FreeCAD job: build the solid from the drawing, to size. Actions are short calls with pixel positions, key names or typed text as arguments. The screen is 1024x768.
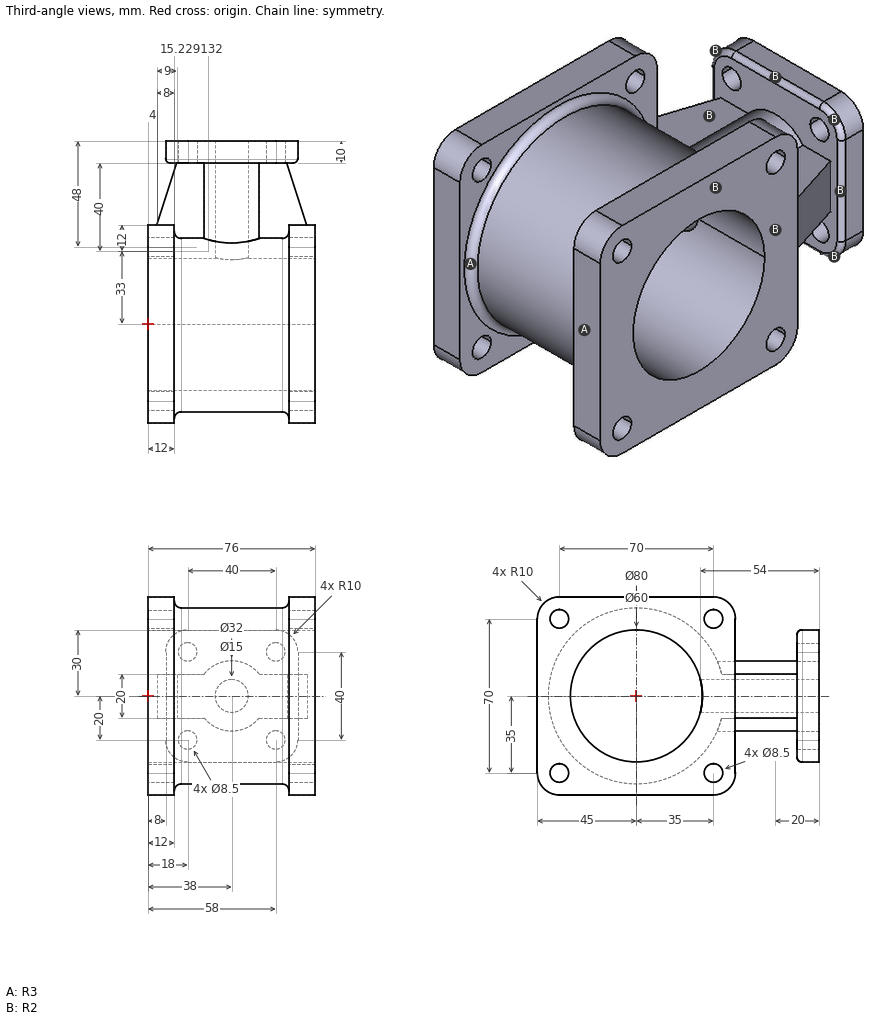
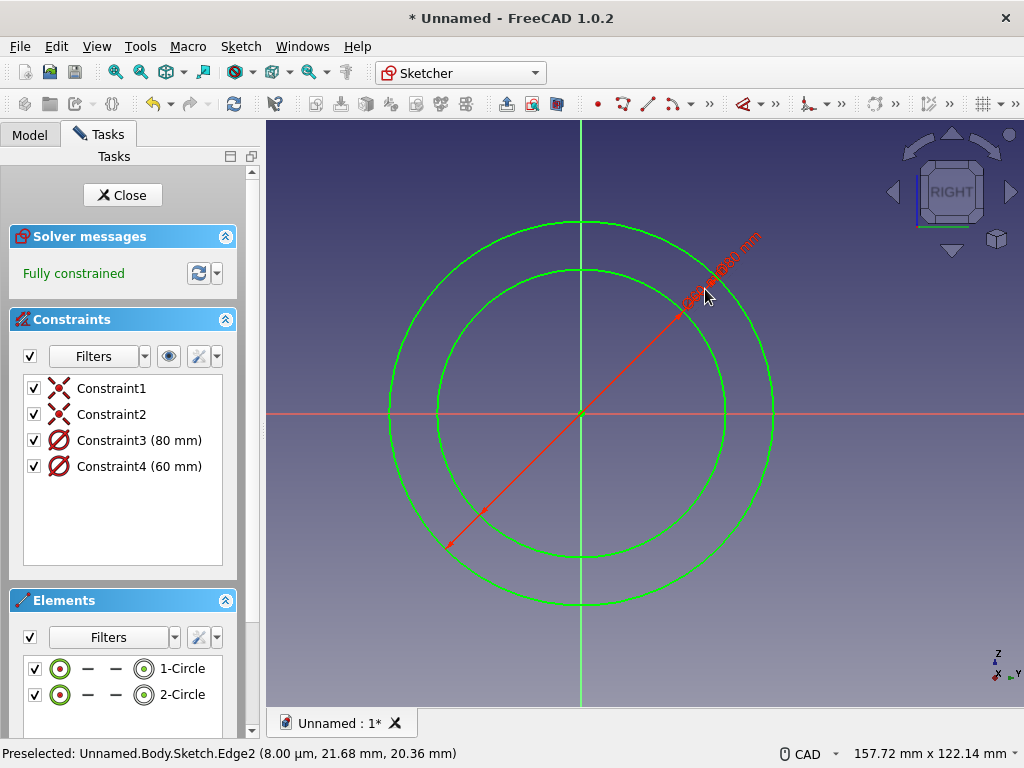
click(123, 195)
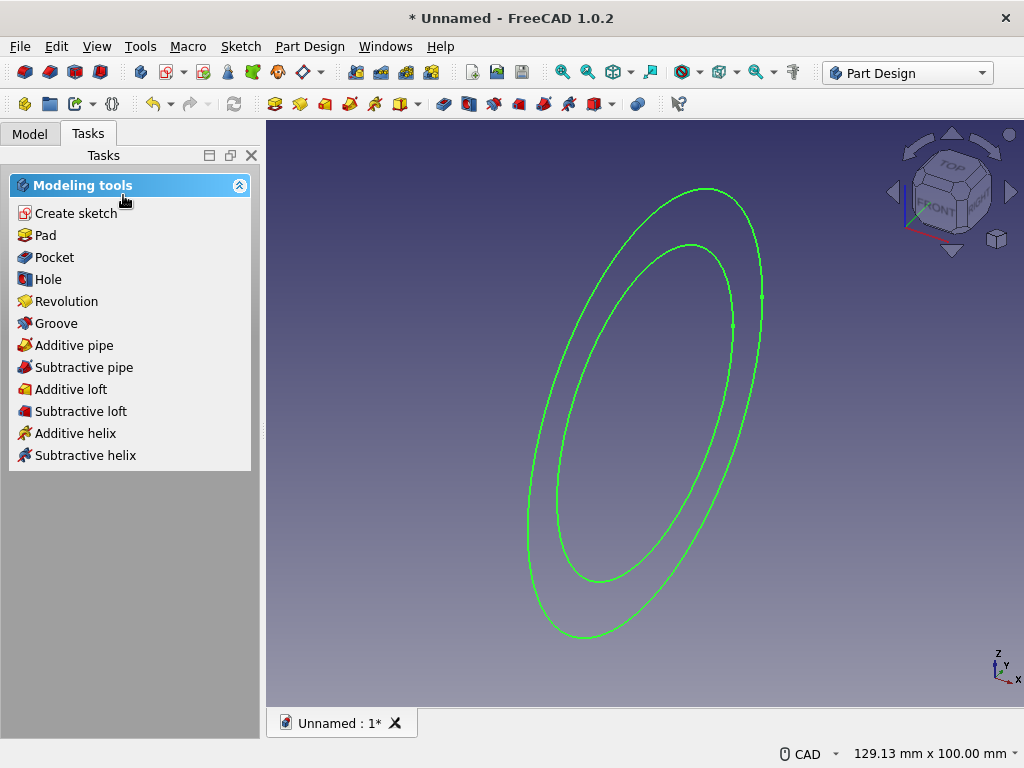
click(275, 104)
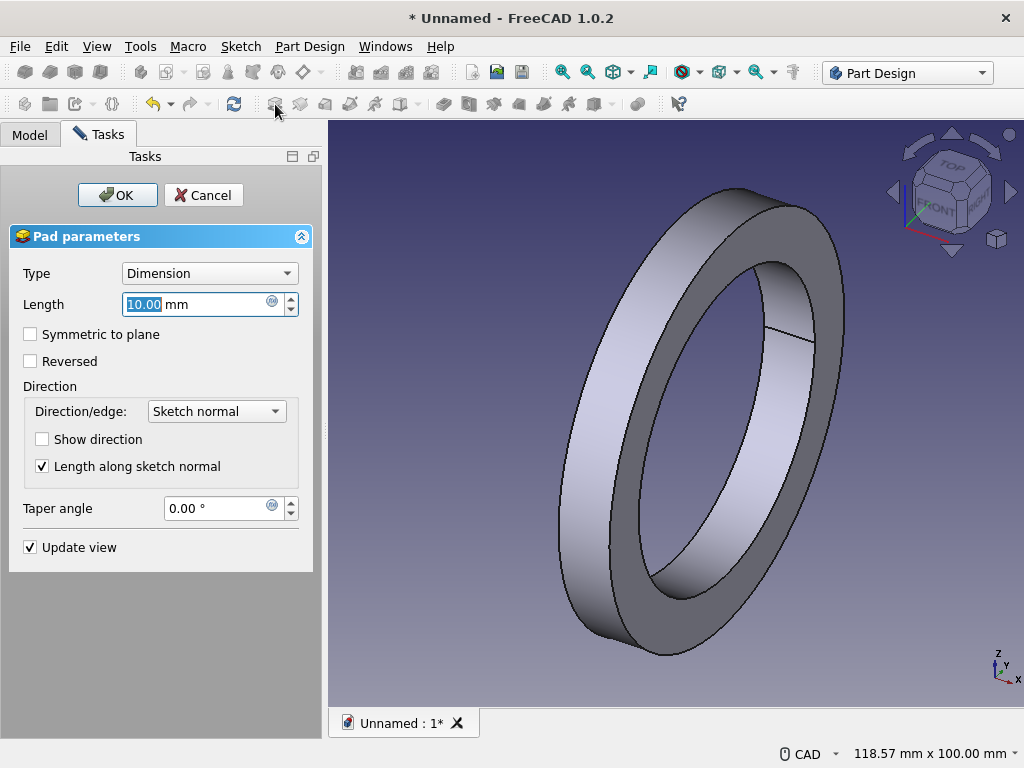
text(76)
key(Tab)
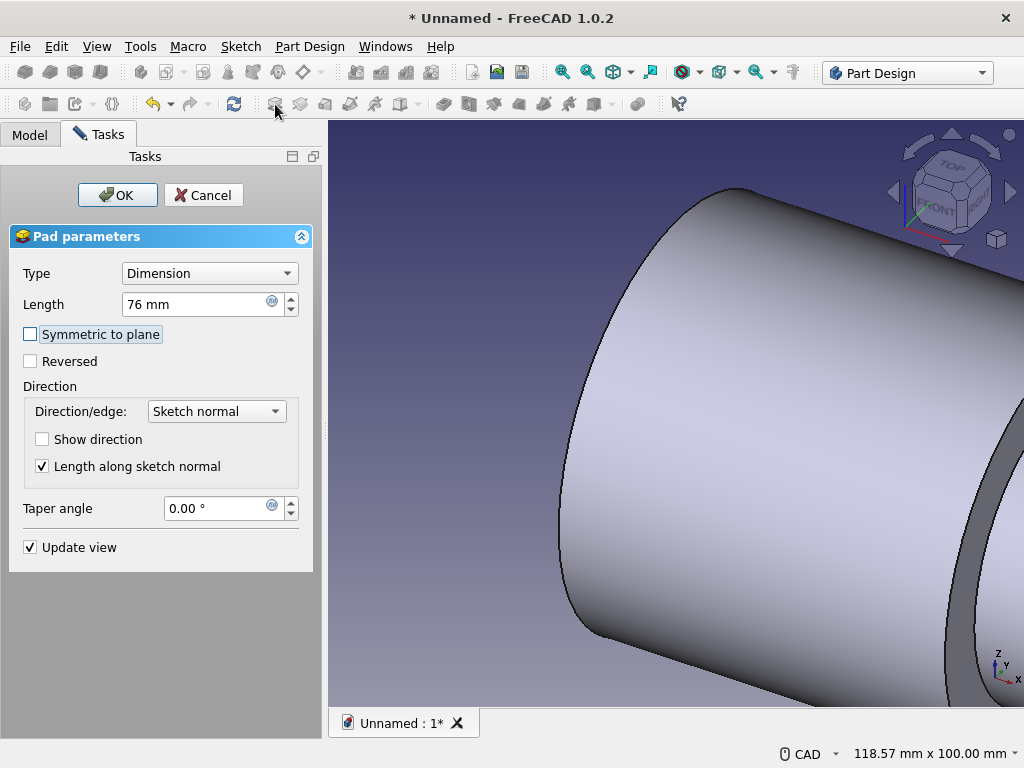
click(118, 195)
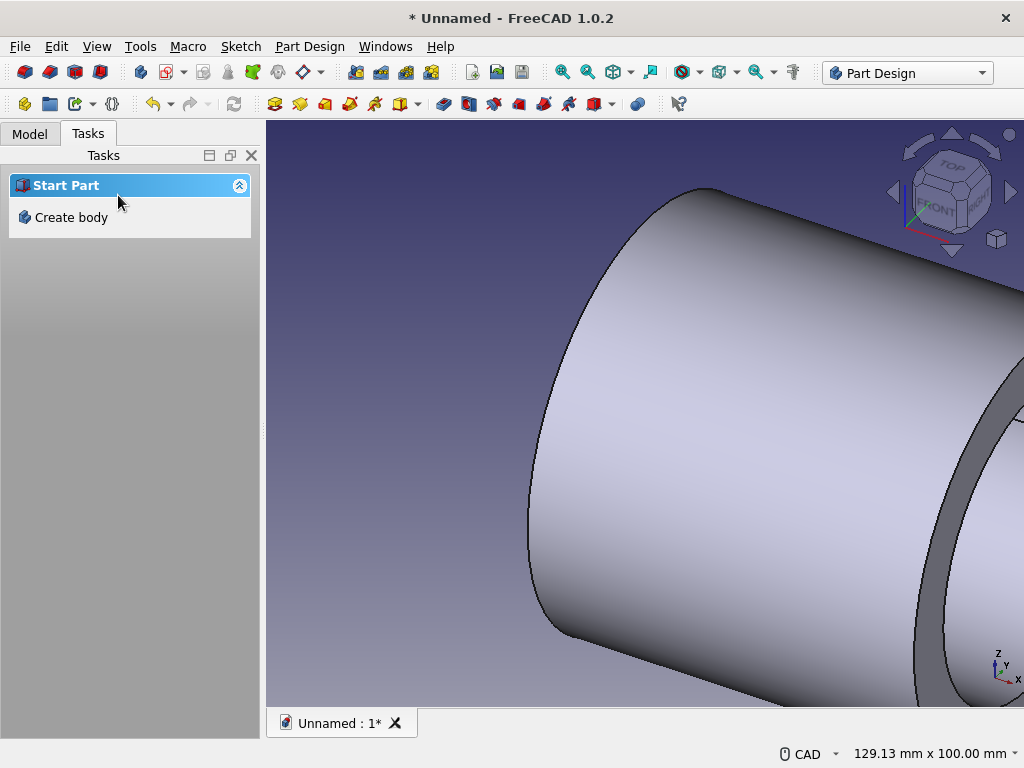
key(v)
key(f)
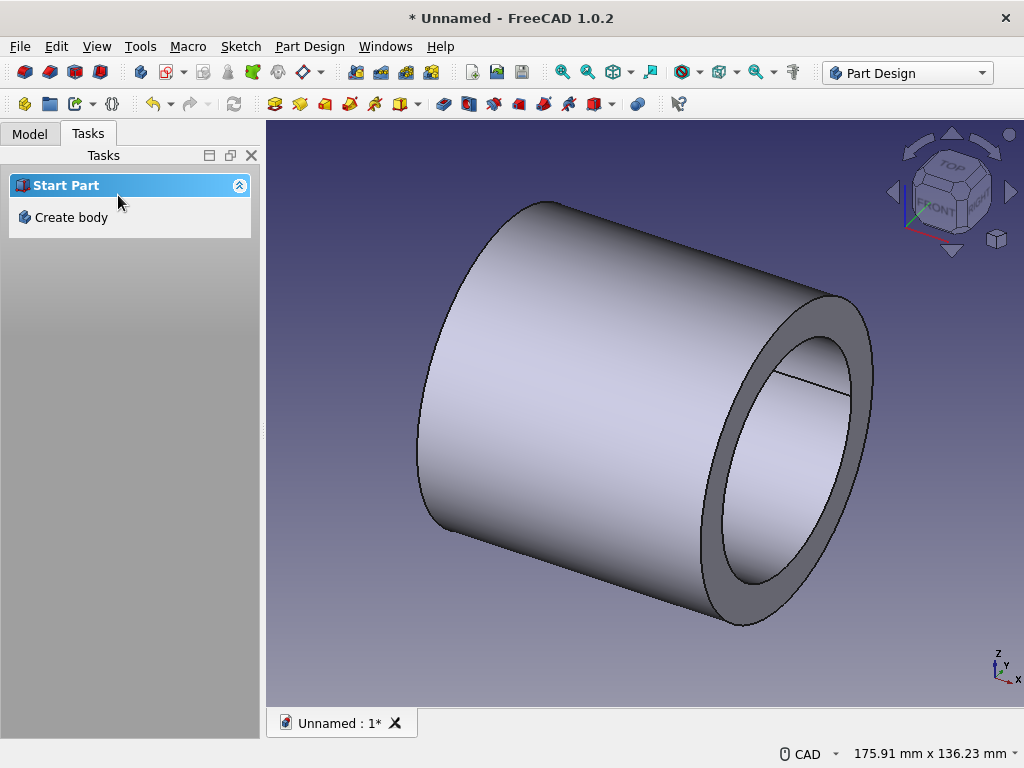
click(166, 72)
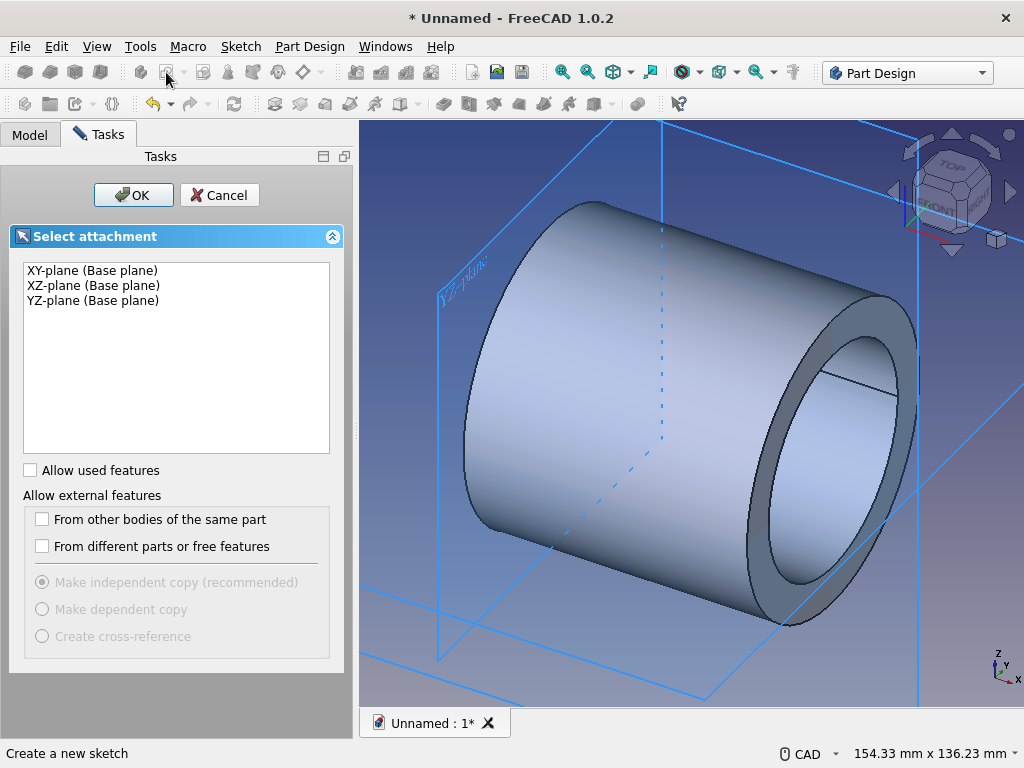
click(84, 300)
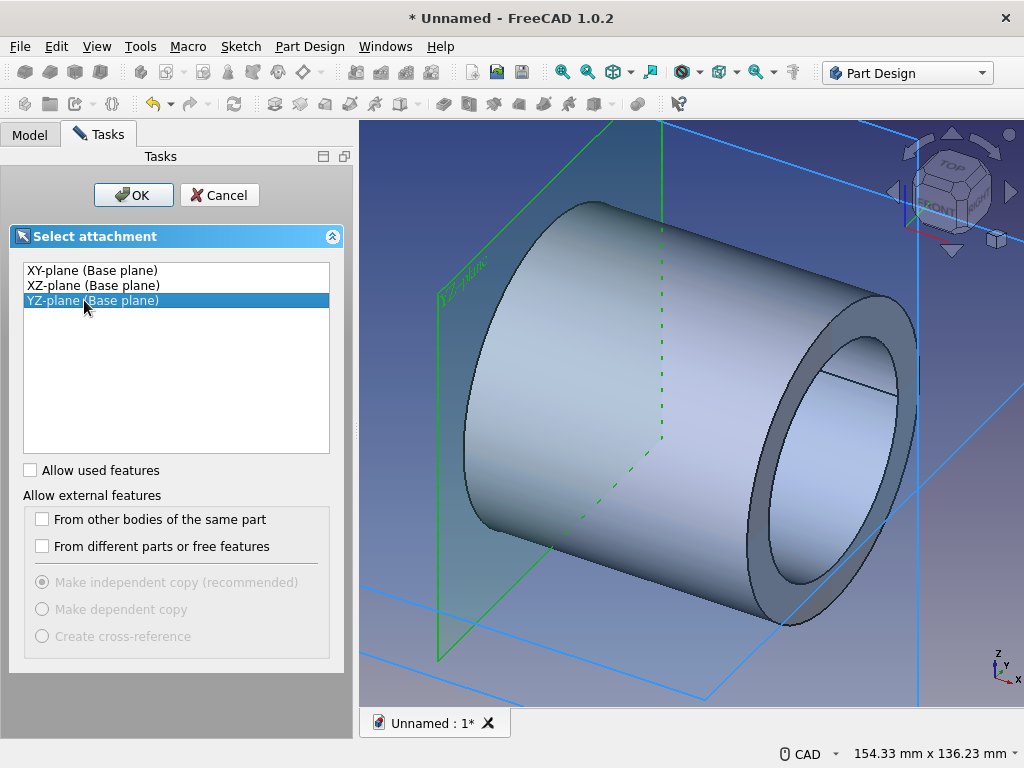
click(134, 195)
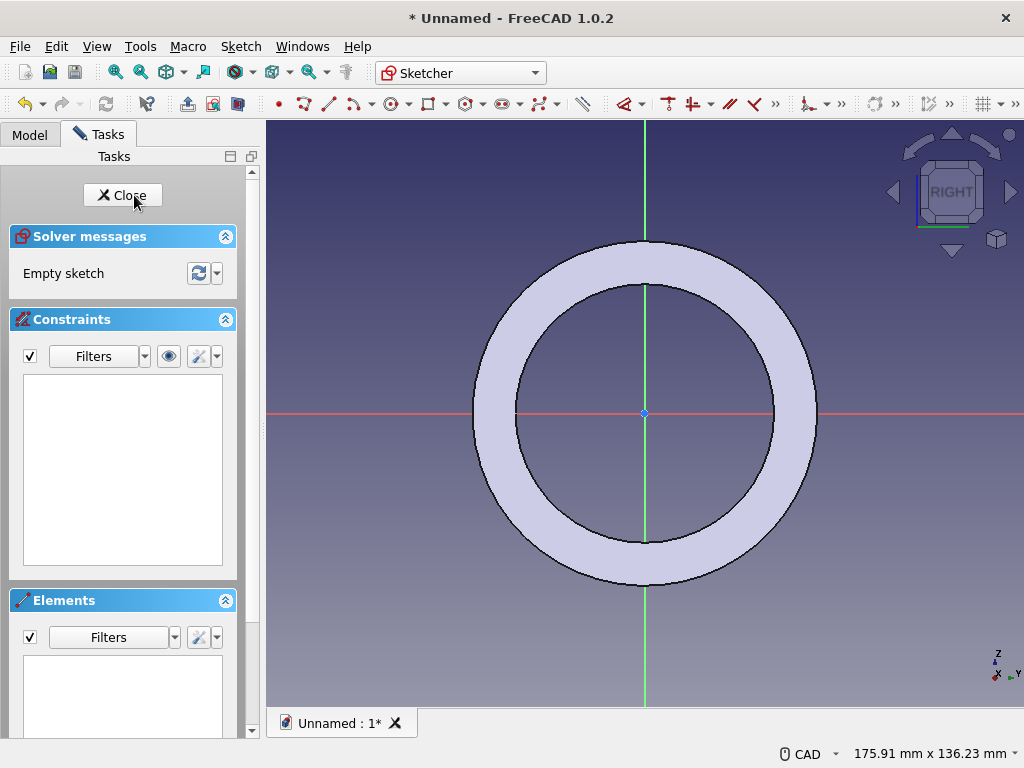
key(q)
key(s)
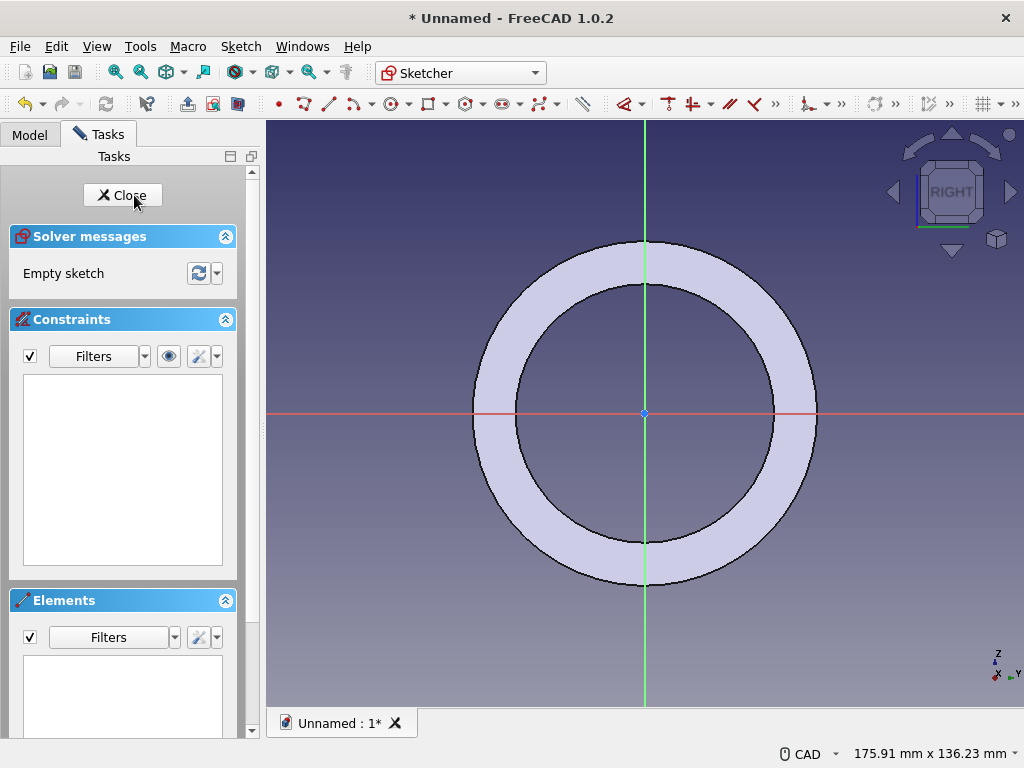
scroll(294, 413, down, 1)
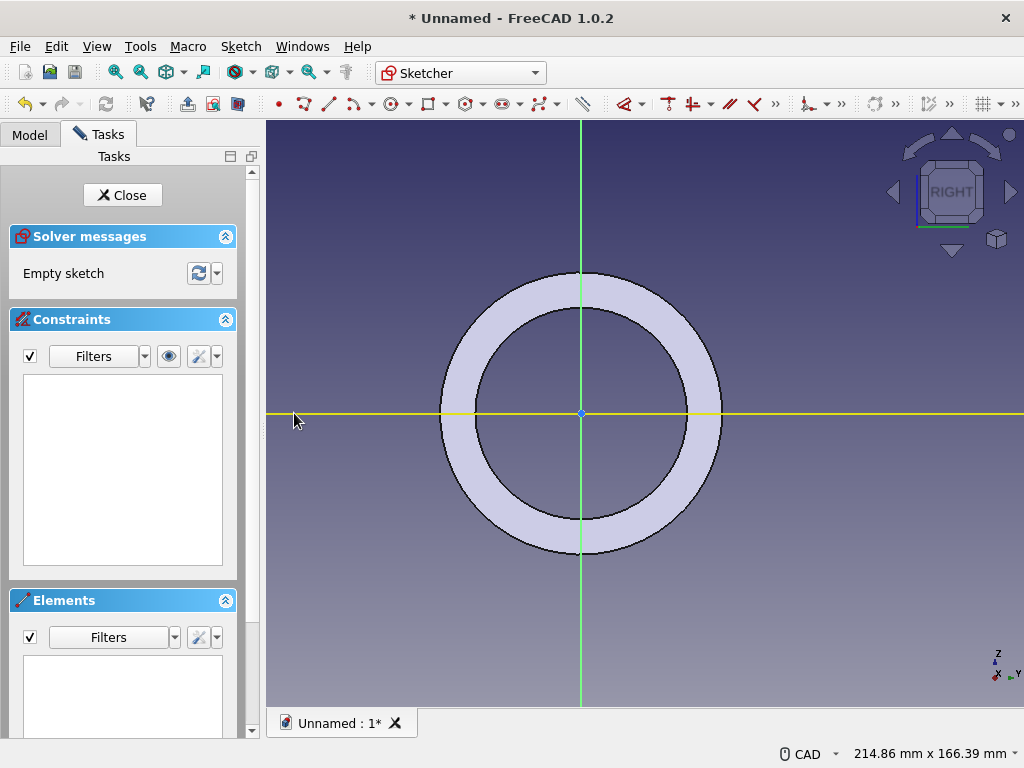
key(g)
key(l)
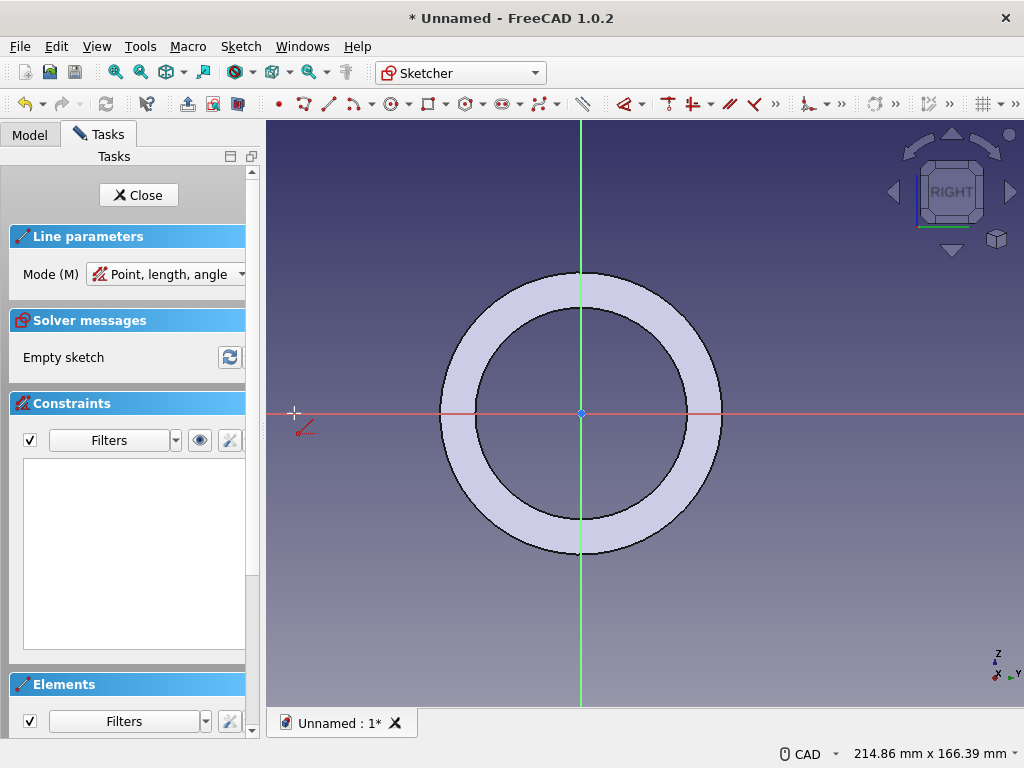
click(422, 537)
click(422, 290)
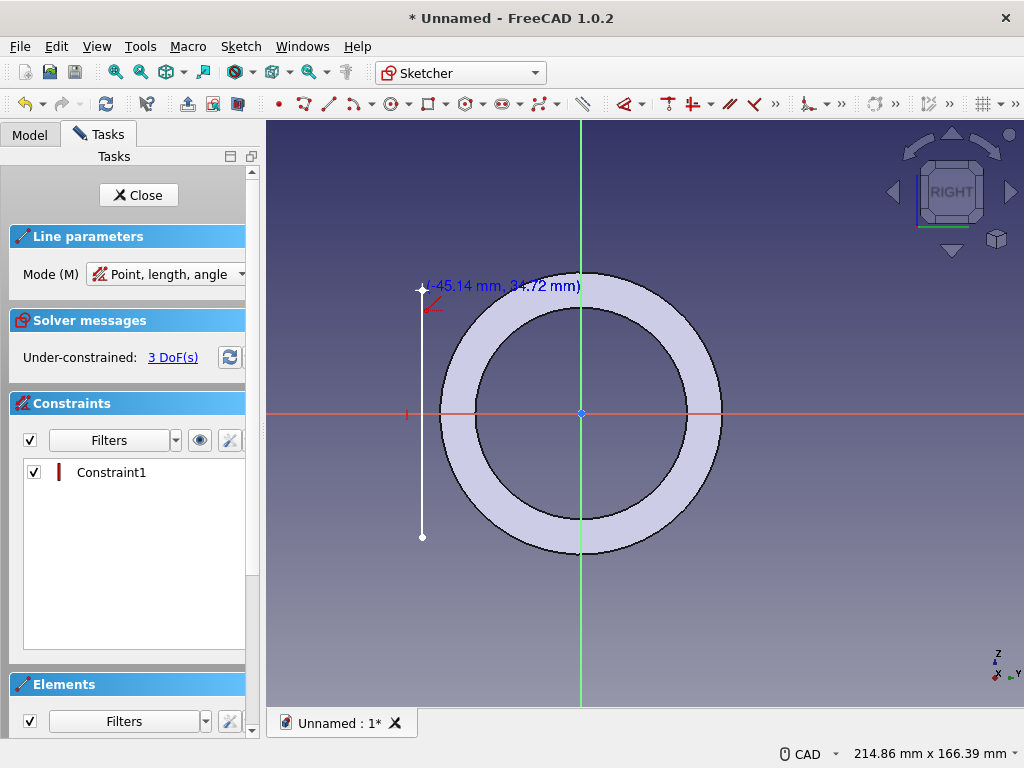
click(458, 255)
click(705, 255)